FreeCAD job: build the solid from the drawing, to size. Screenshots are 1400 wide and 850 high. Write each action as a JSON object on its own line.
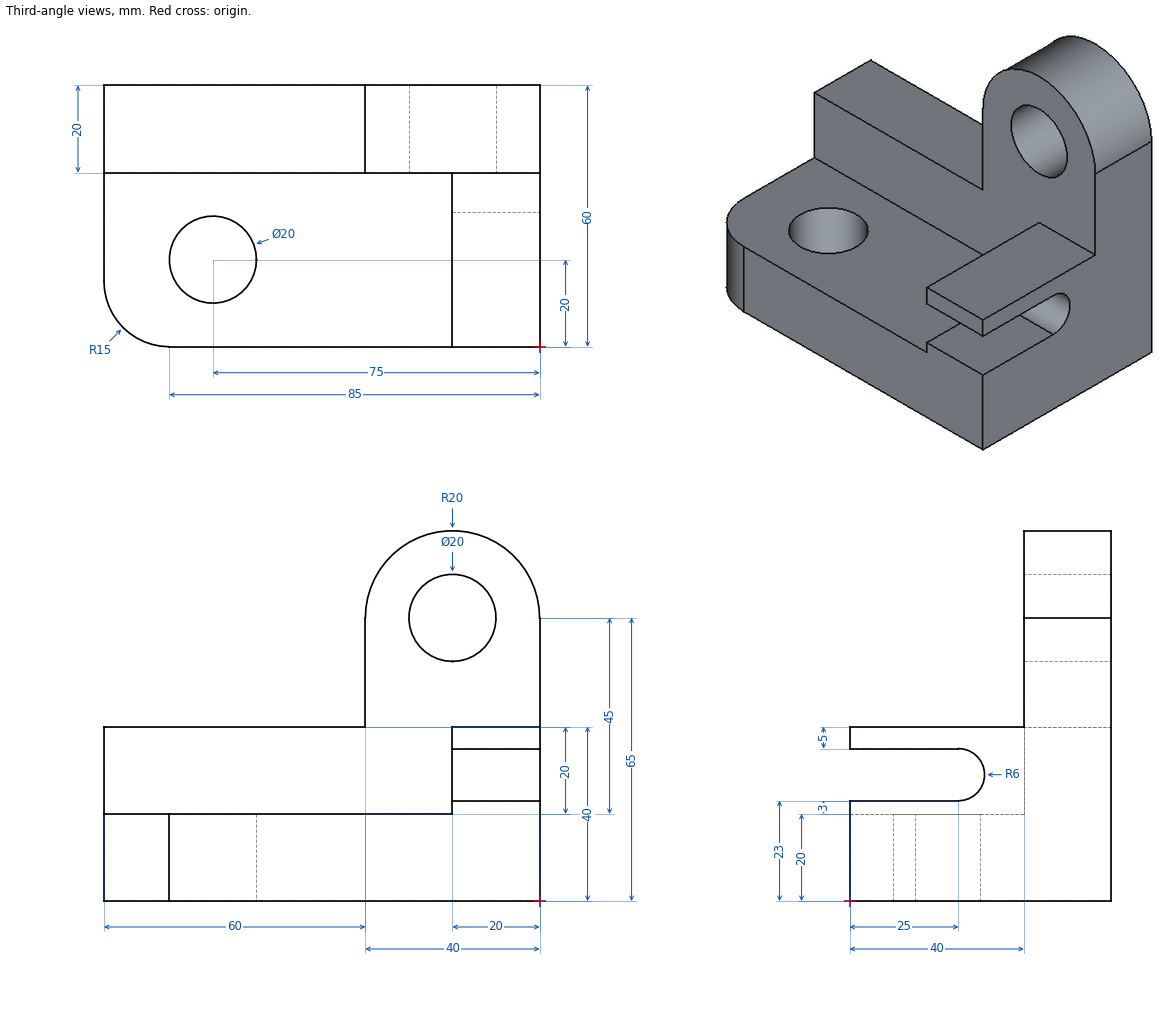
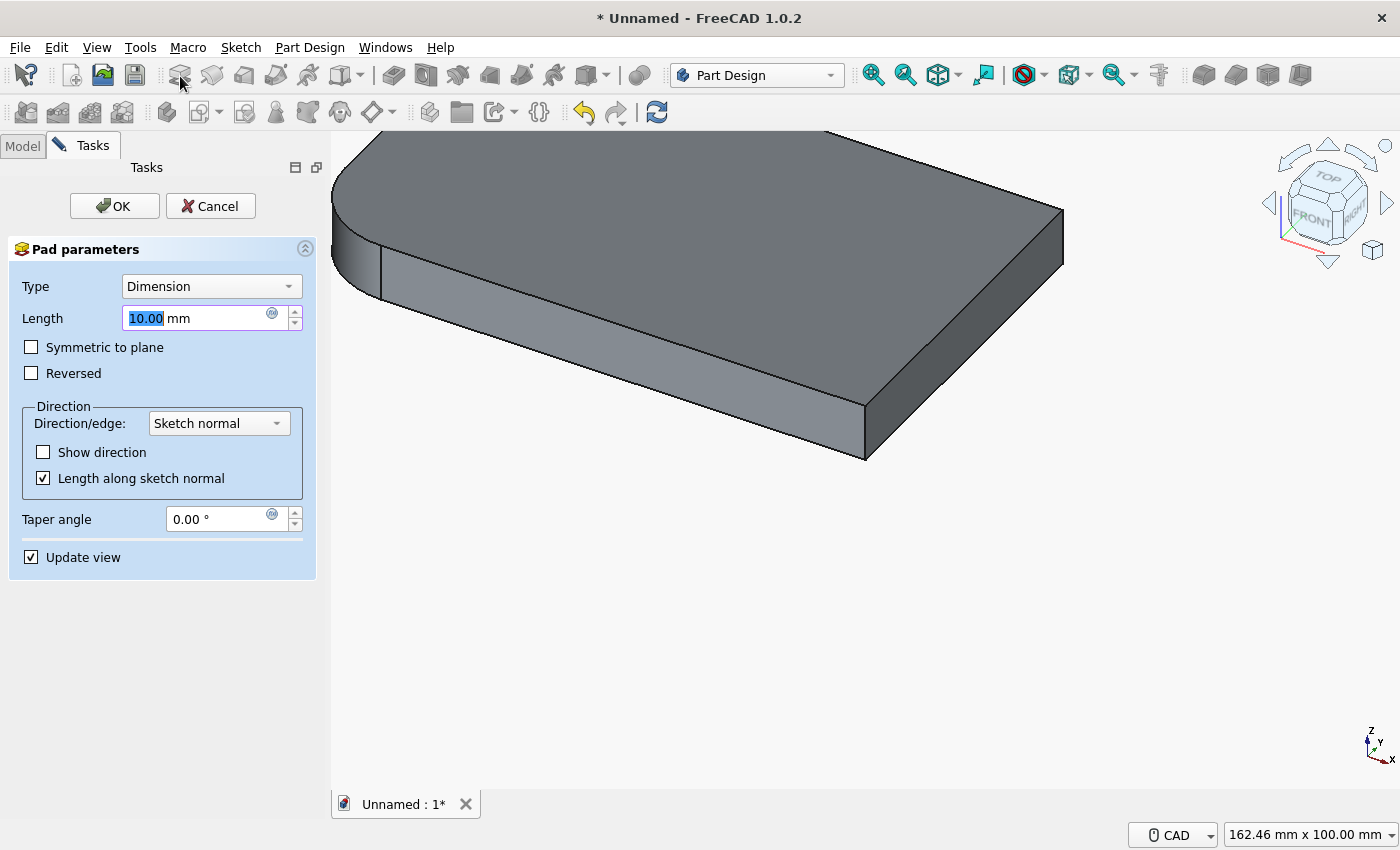
{"action": "type", "text": "20"}
{"action": "key", "text": "Tab"}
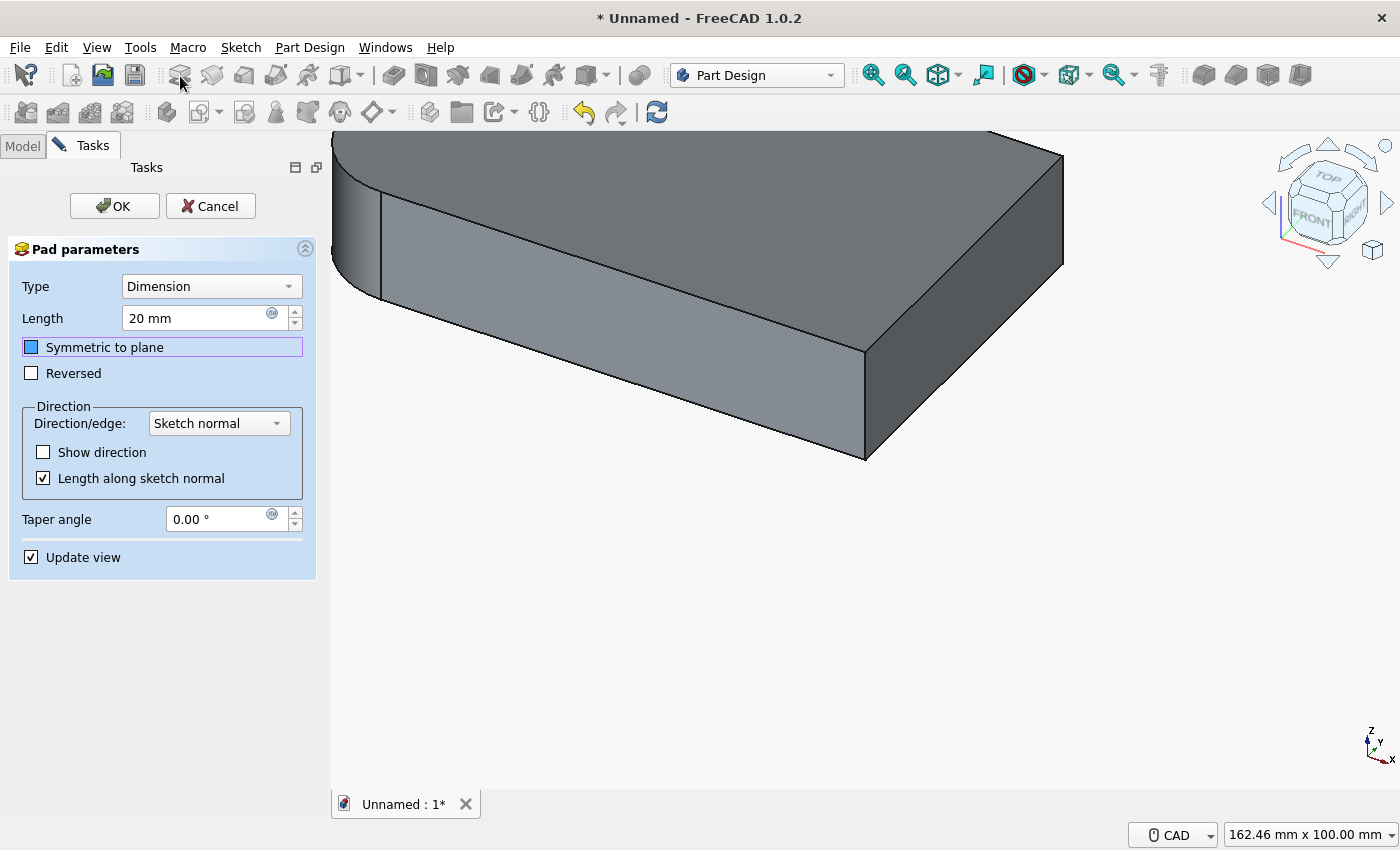
{"action": "left_click", "coordinate": [115, 206]}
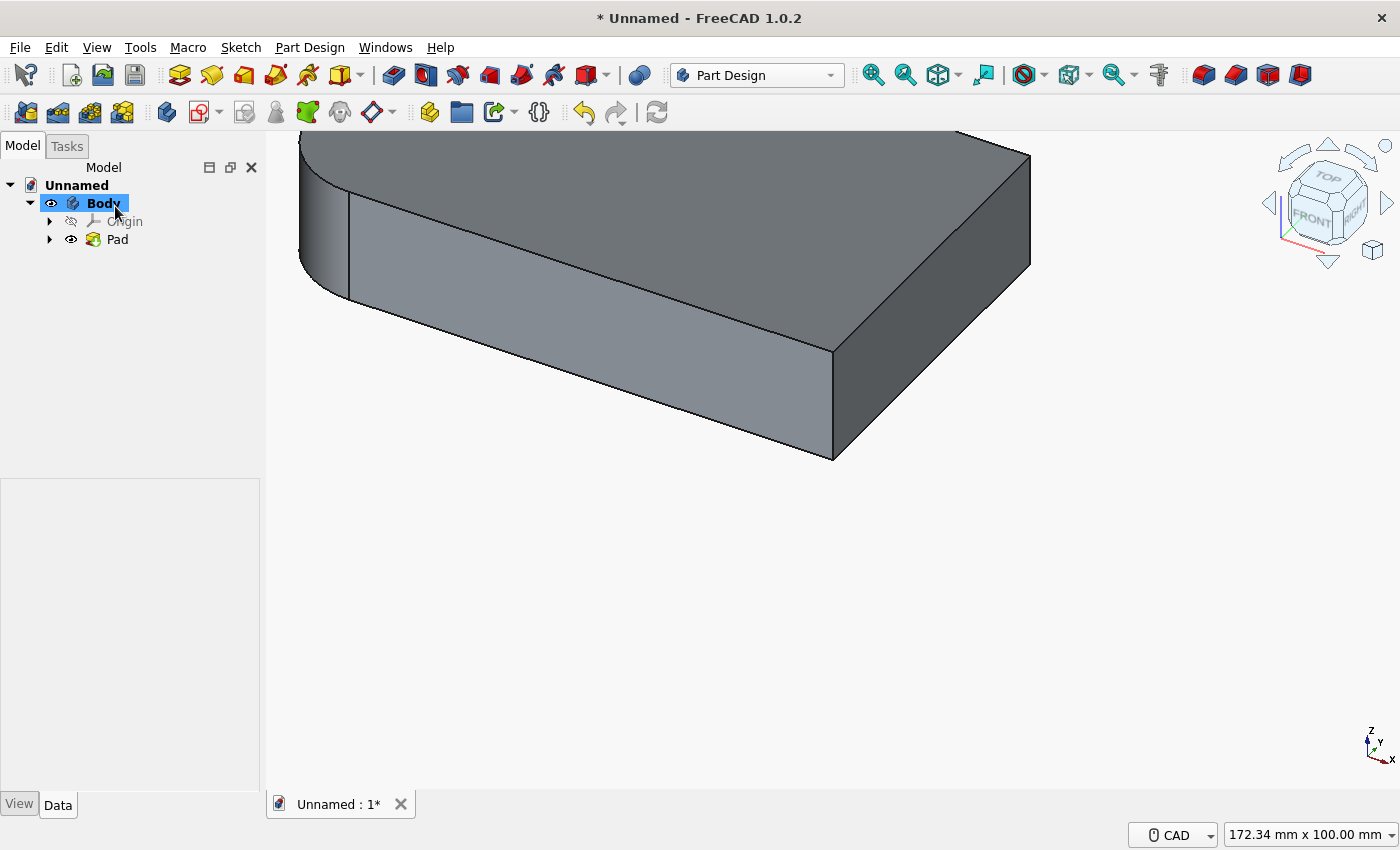
{"action": "left_click", "coordinate": [874, 76]}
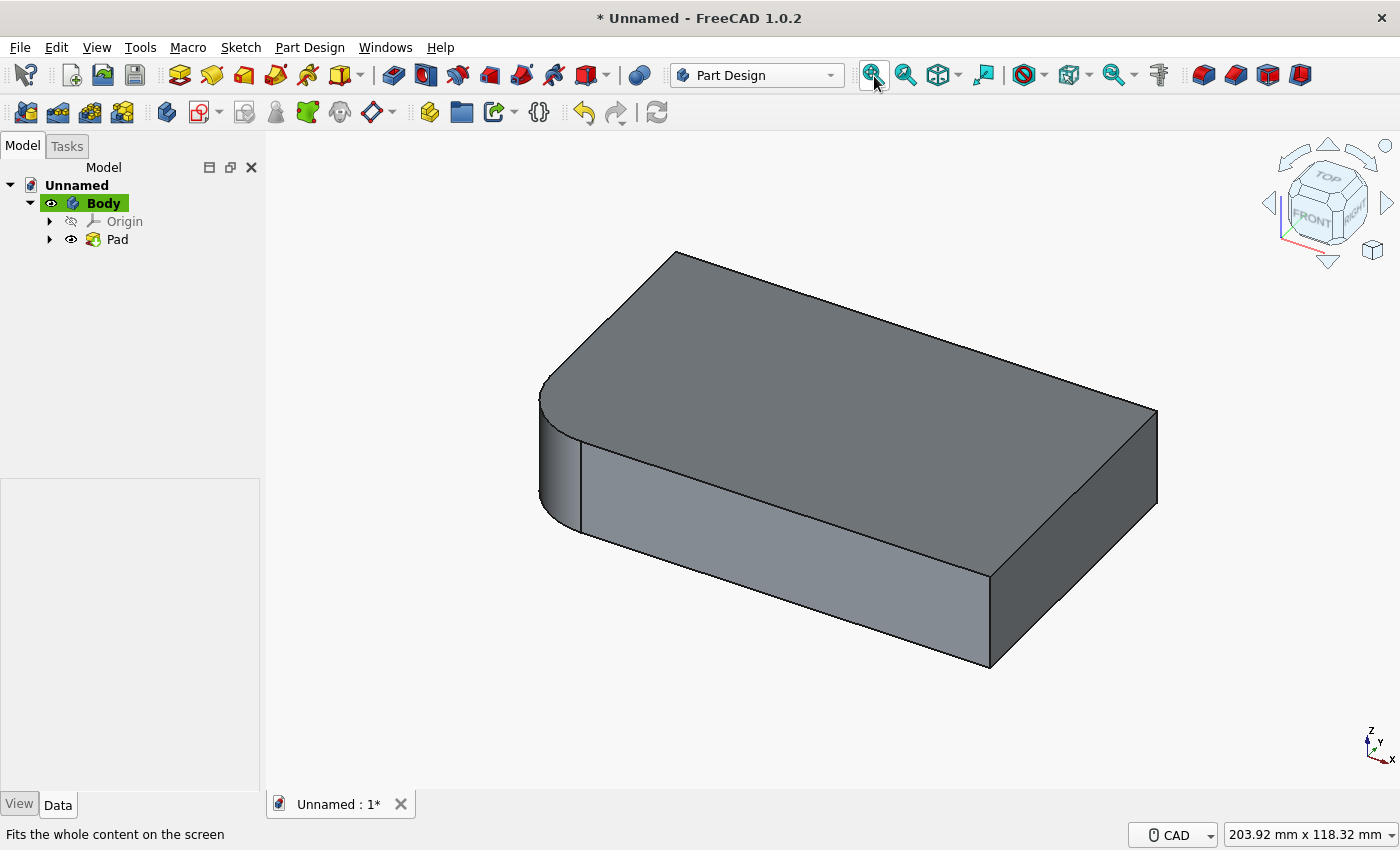
{"action": "left_click", "coordinate": [1121, 491]}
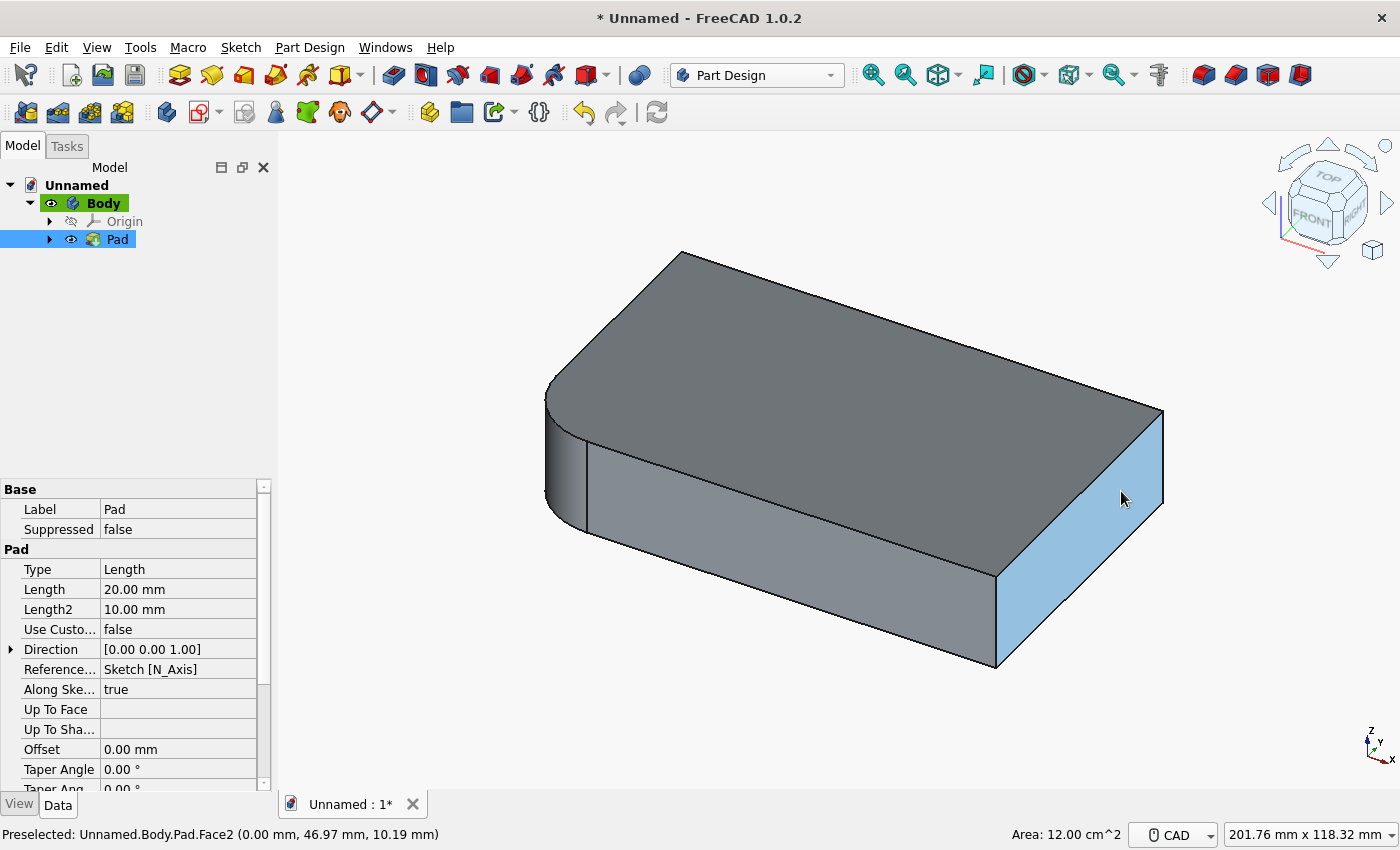
{"action": "left_click", "coordinate": [200, 112]}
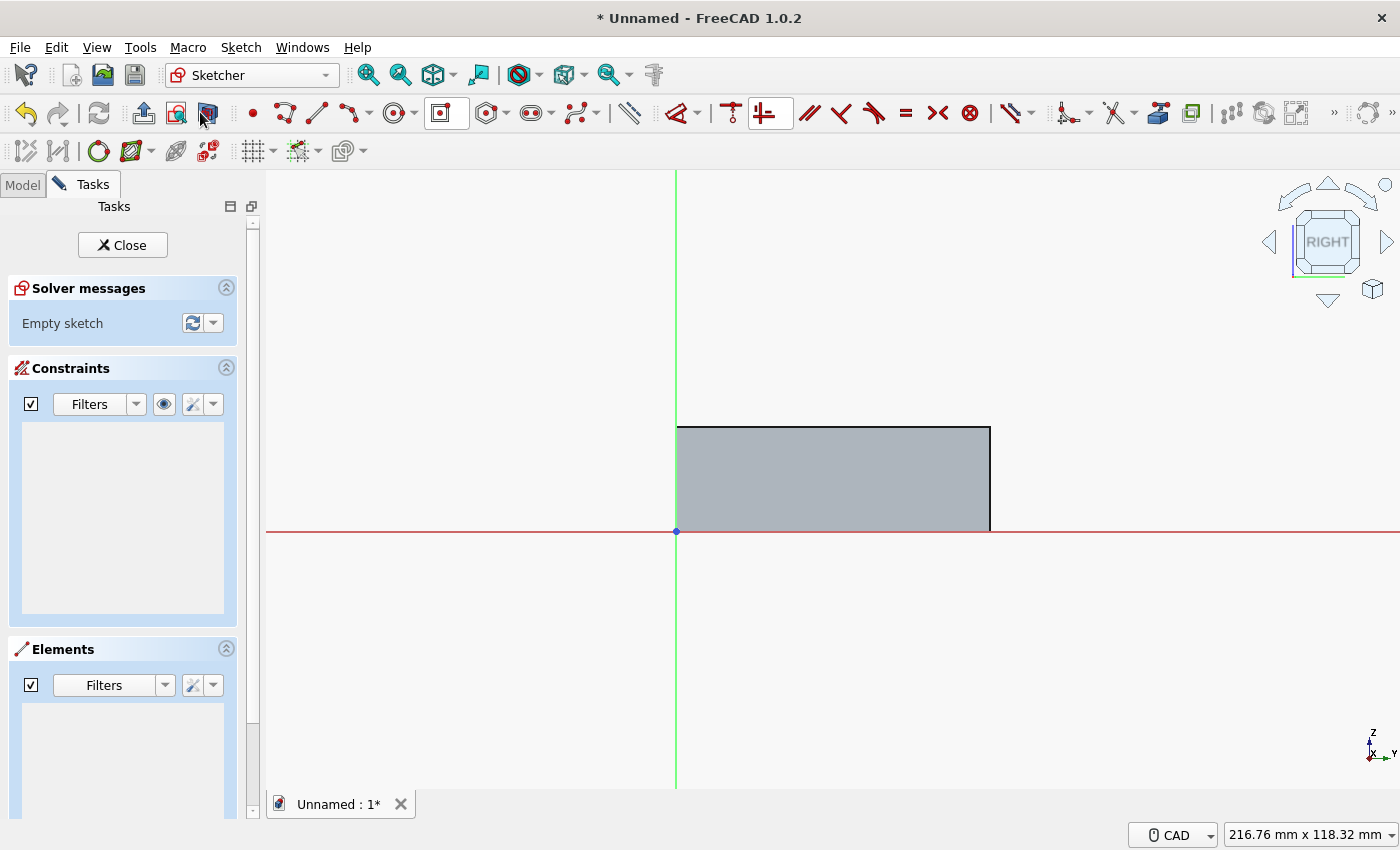
{"action": "scroll", "coordinate": [800, 364], "scroll_direction": "up", "scroll_amount": 3}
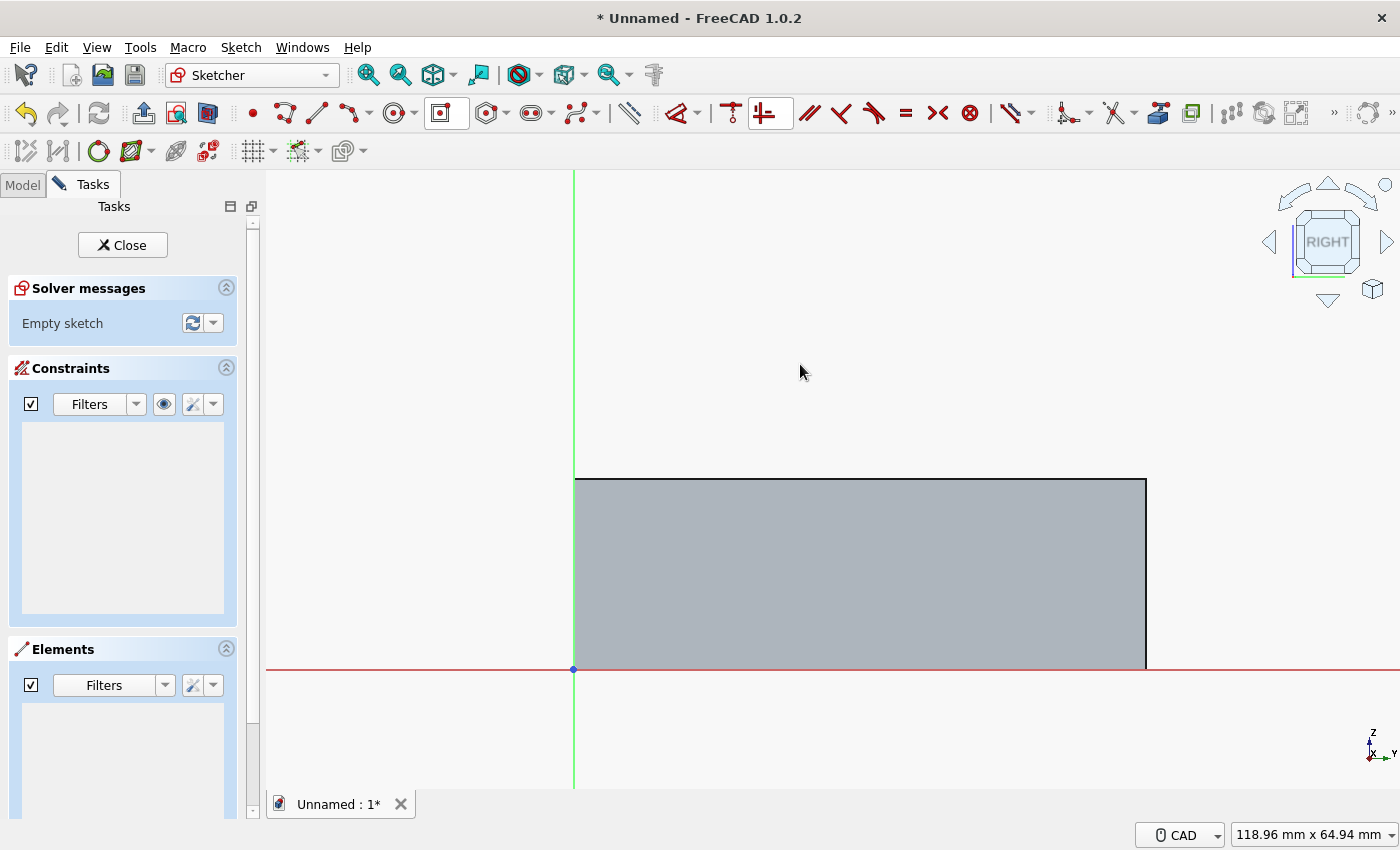
{"action": "key", "text": "g m"}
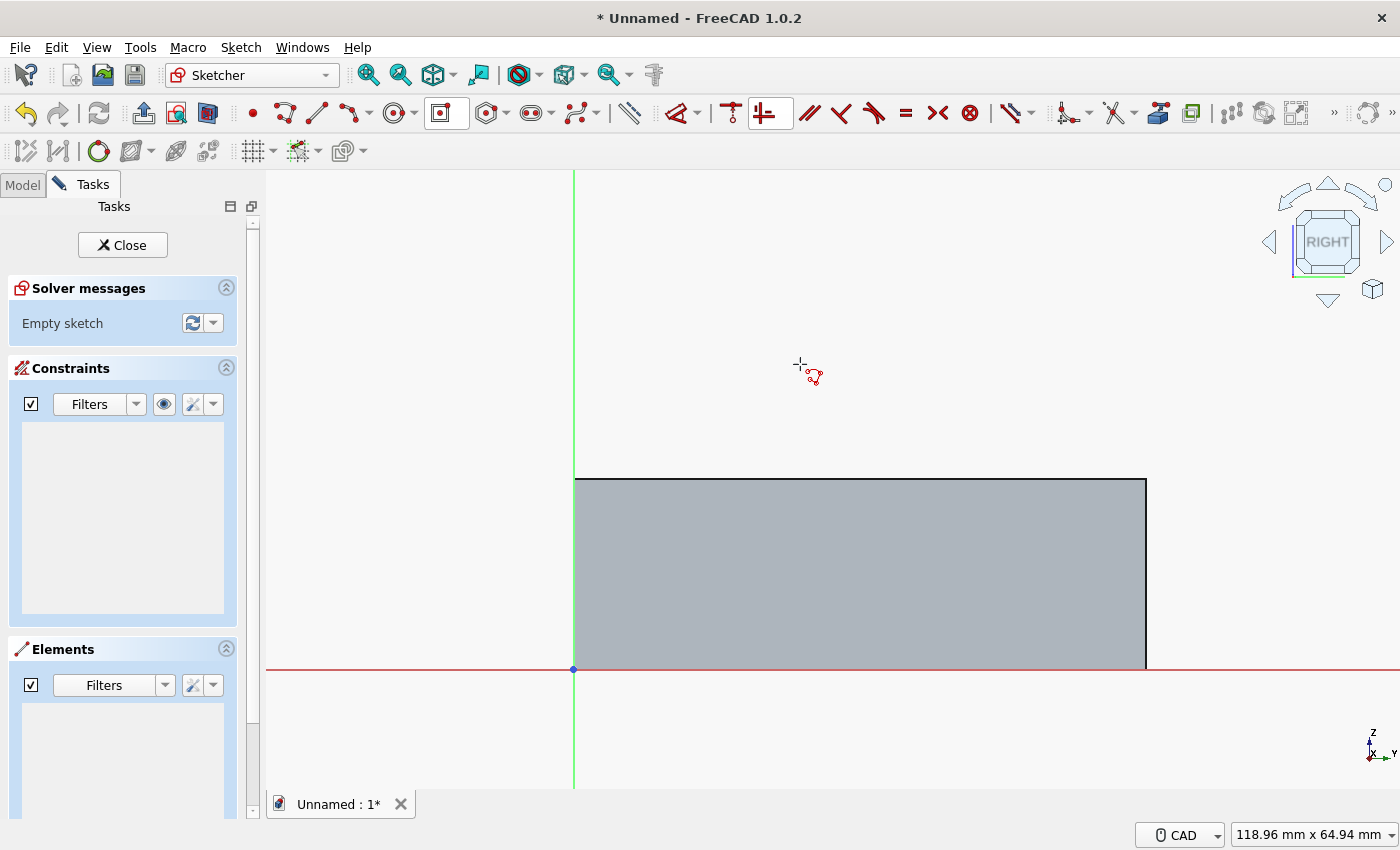
{"action": "left_click", "coordinate": [812, 450]}
{"action": "left_click", "coordinate": [574, 450]}
{"action": "left_click", "coordinate": [583, 479]}
{"action": "left_click", "coordinate": [955, 479]}
{"action": "left_click", "coordinate": [955, 288]}
{"action": "left_click", "coordinate": [574, 288]}
{"action": "left_click", "coordinate": [583, 336]}
{"action": "left_click", "coordinate": [812, 336]}
{"action": "right_click", "coordinate": [812, 336]}